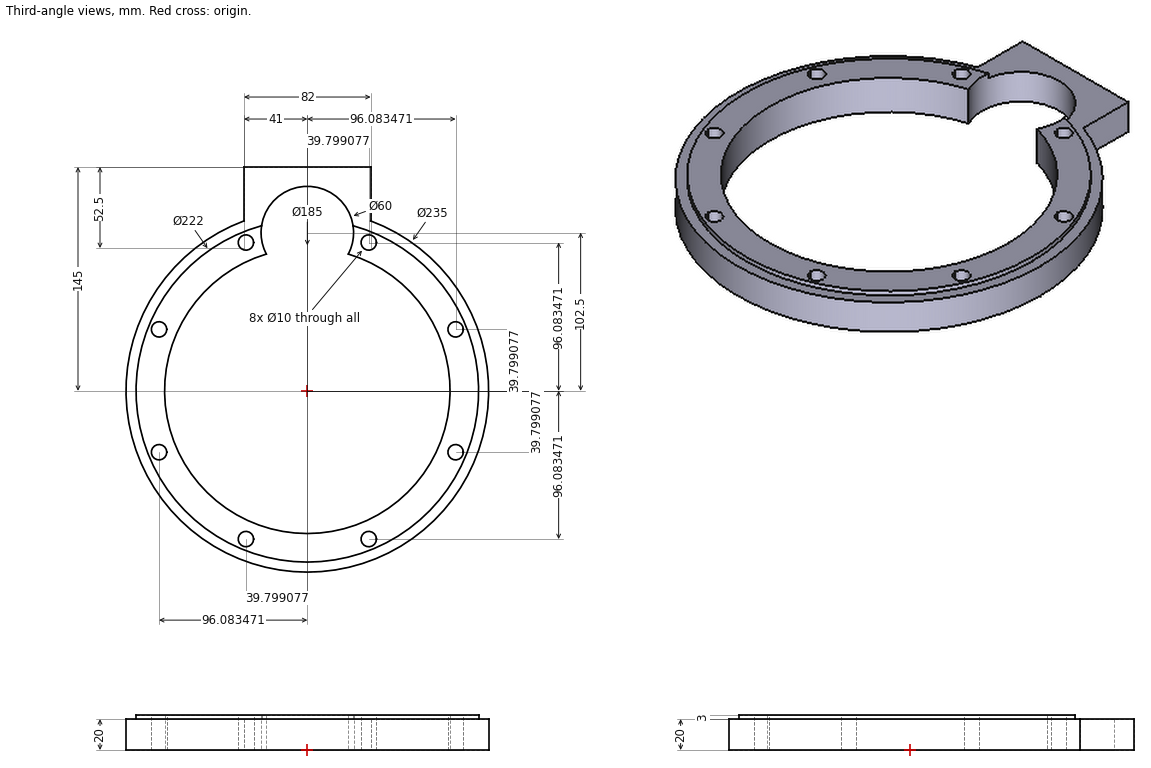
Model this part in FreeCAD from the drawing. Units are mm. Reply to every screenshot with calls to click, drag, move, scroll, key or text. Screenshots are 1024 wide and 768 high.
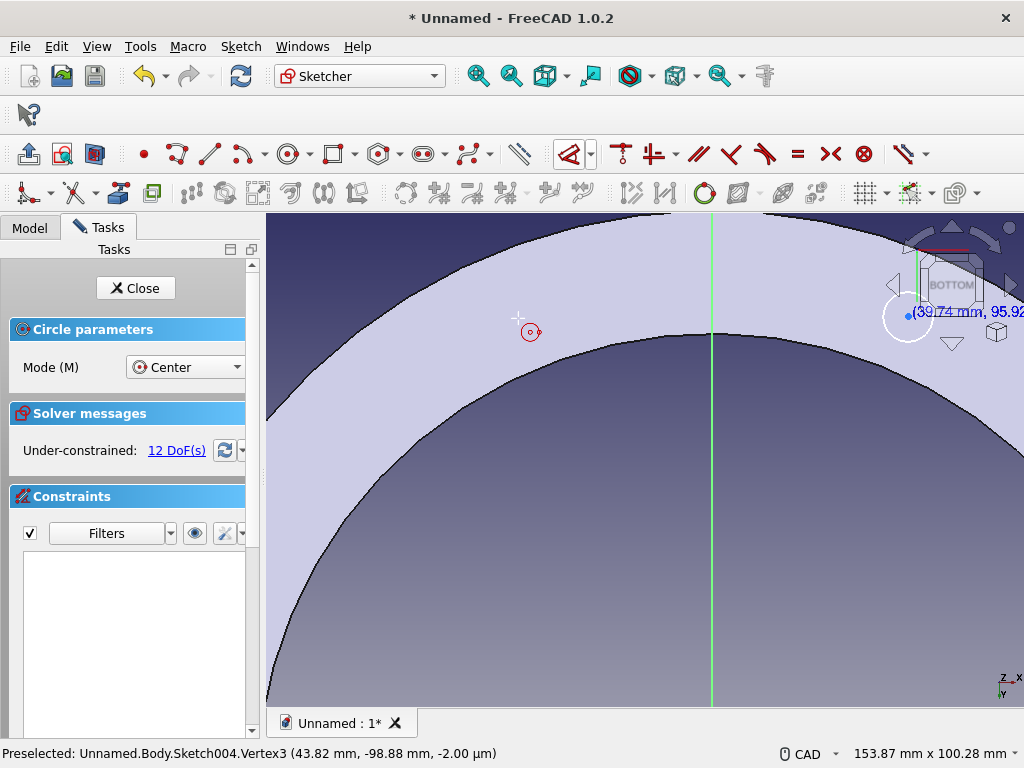
click(516, 316)
click(534, 299)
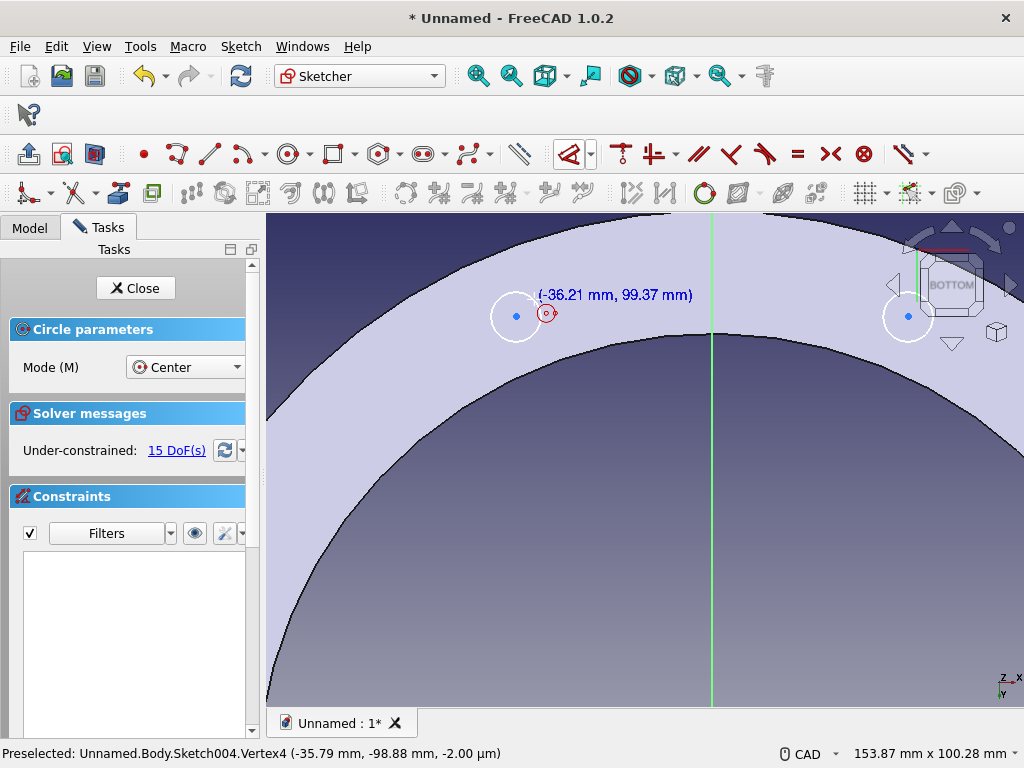
scroll(518, 318, down, 6)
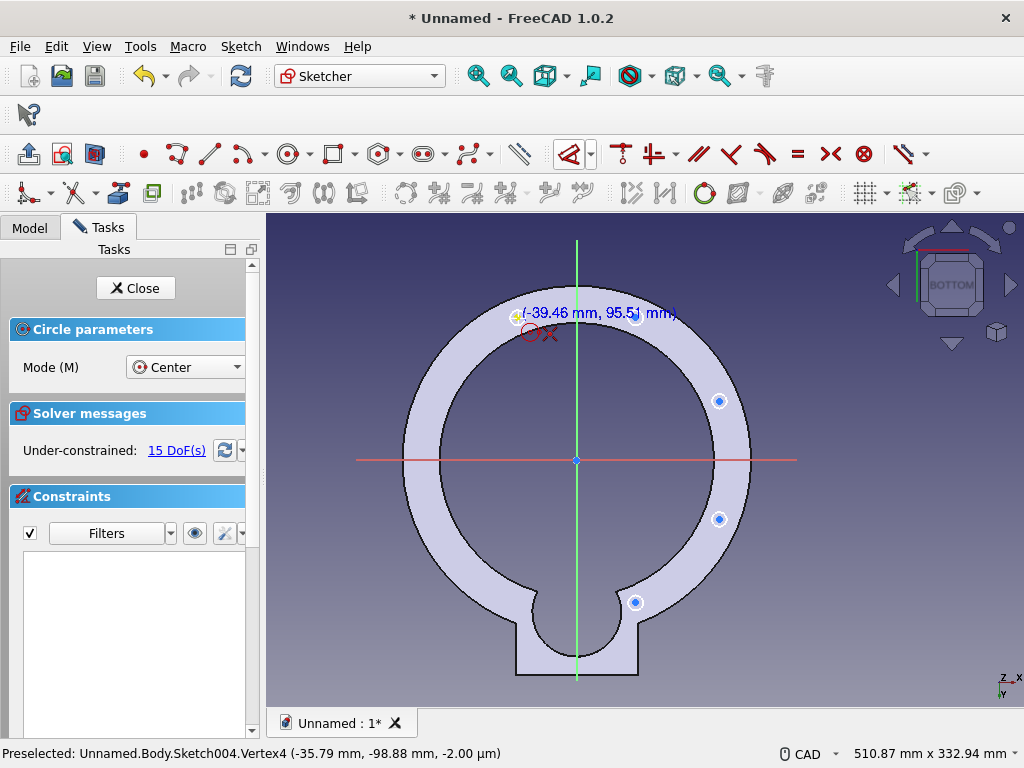
scroll(434, 401, up, 6)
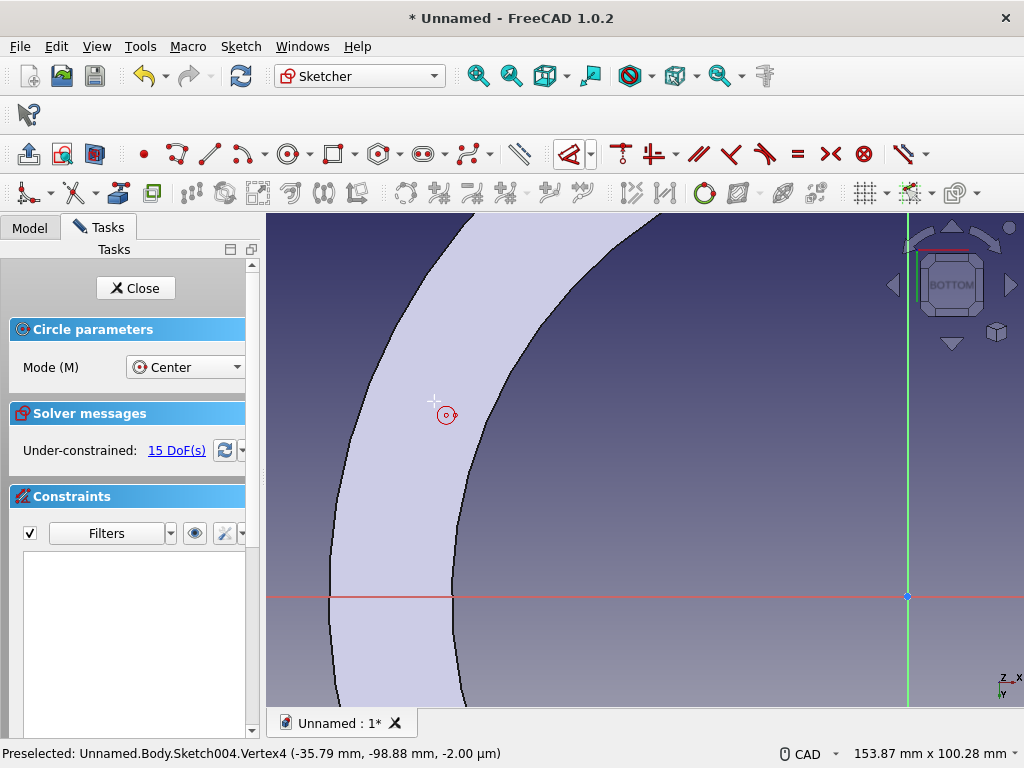
click(434, 400)
click(452, 383)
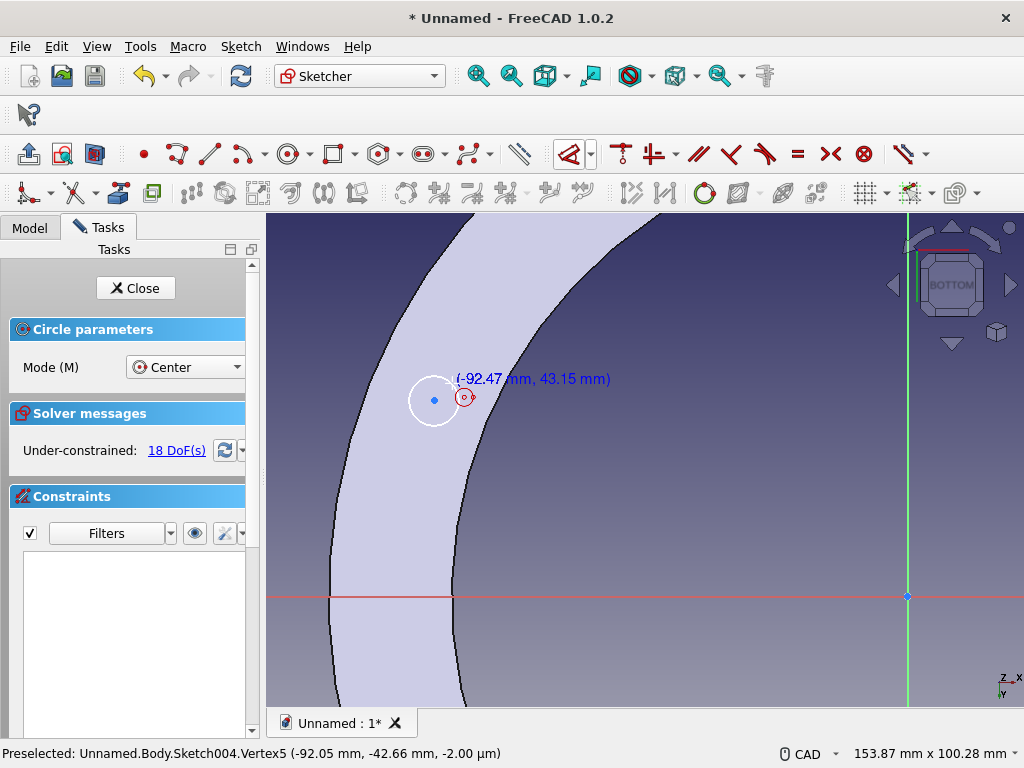
scroll(434, 401, down, 6)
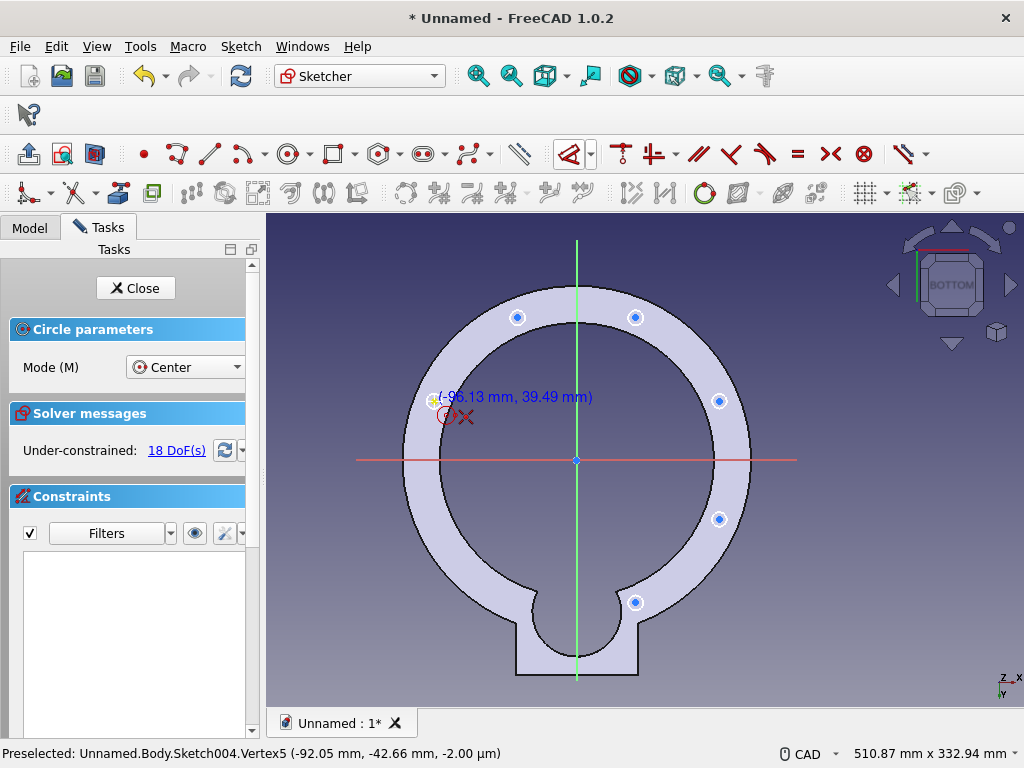
scroll(434, 519, up, 6)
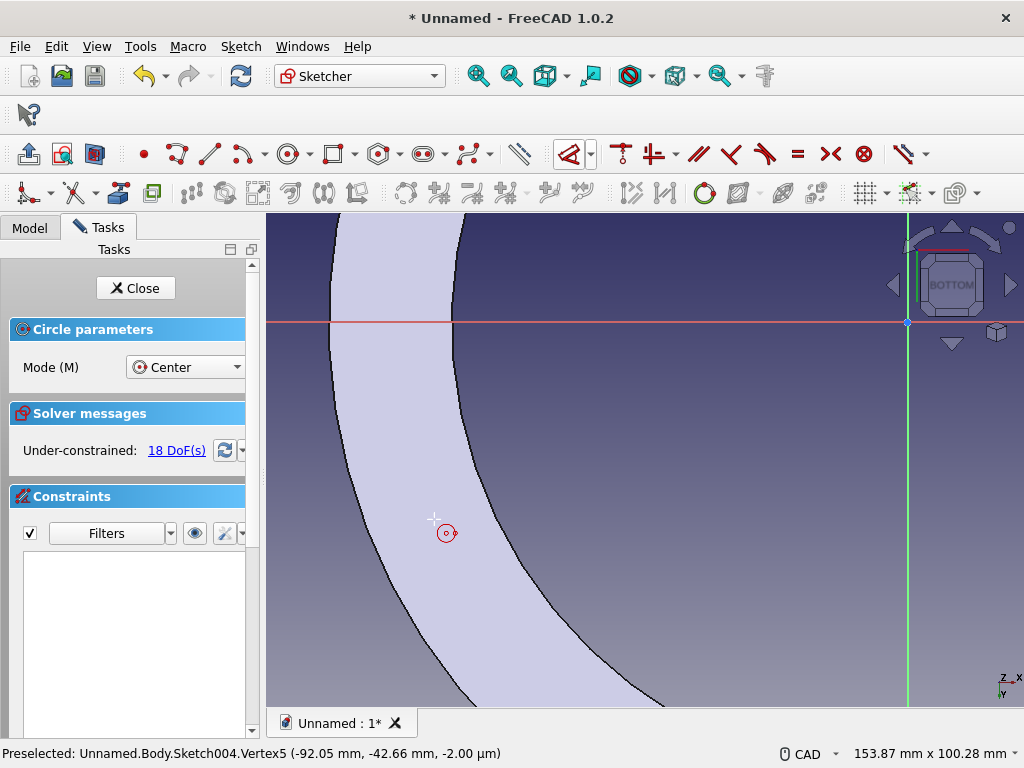
click(434, 518)
click(452, 501)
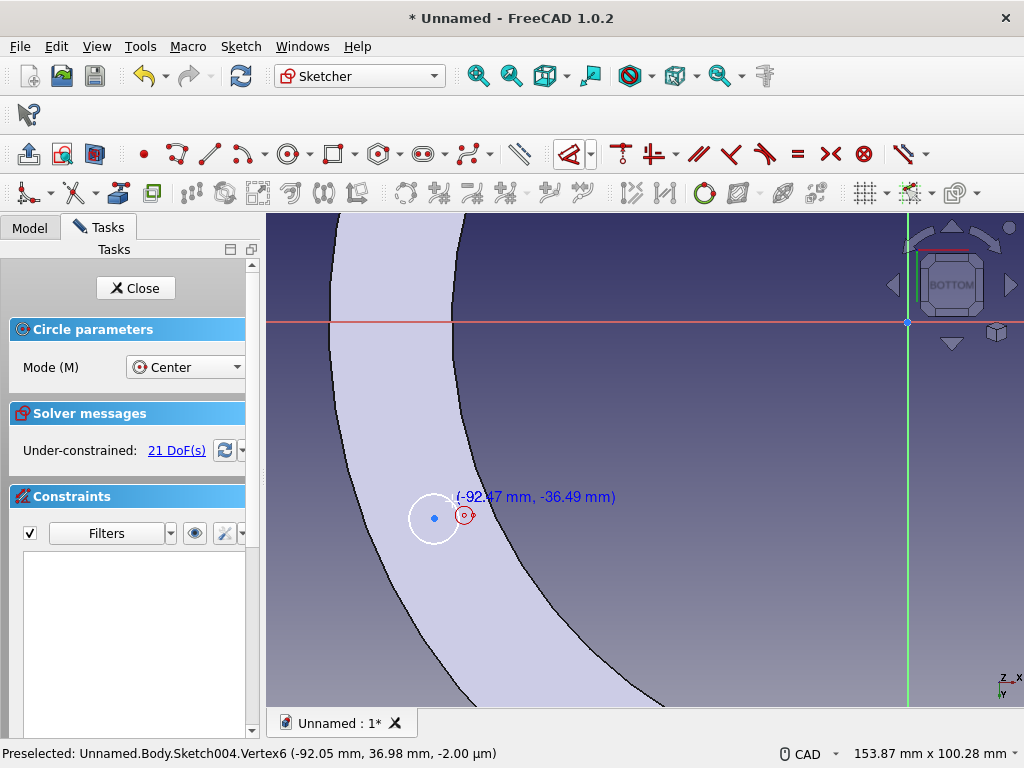
scroll(434, 519, down, 6)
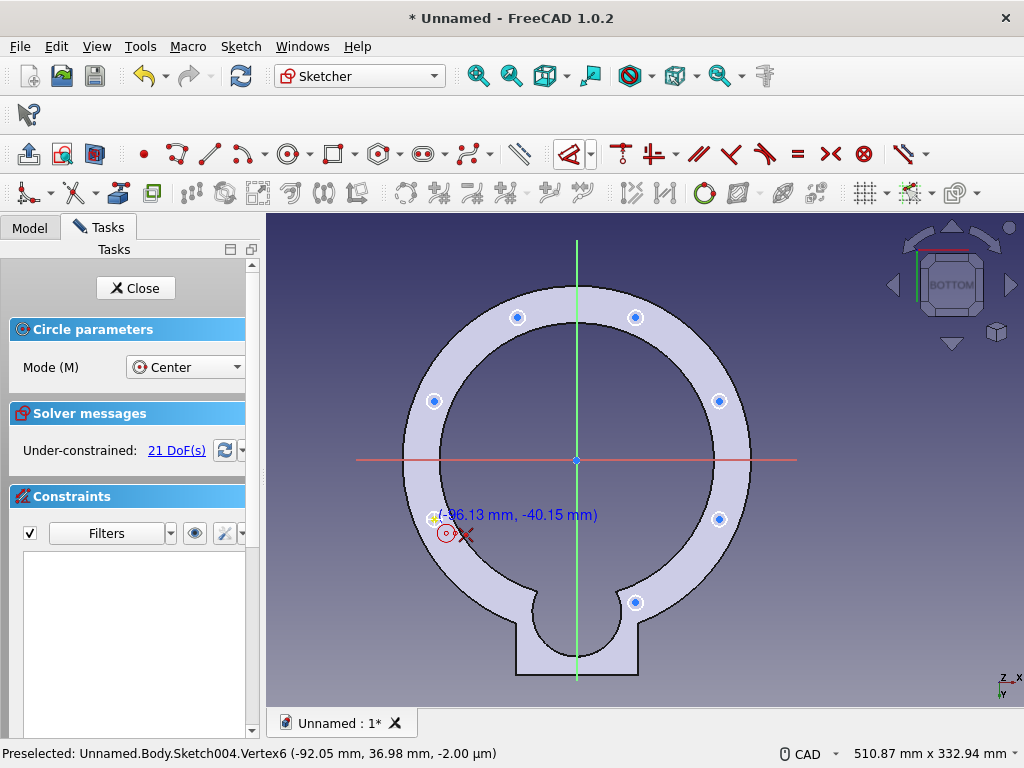
scroll(518, 603, up, 6)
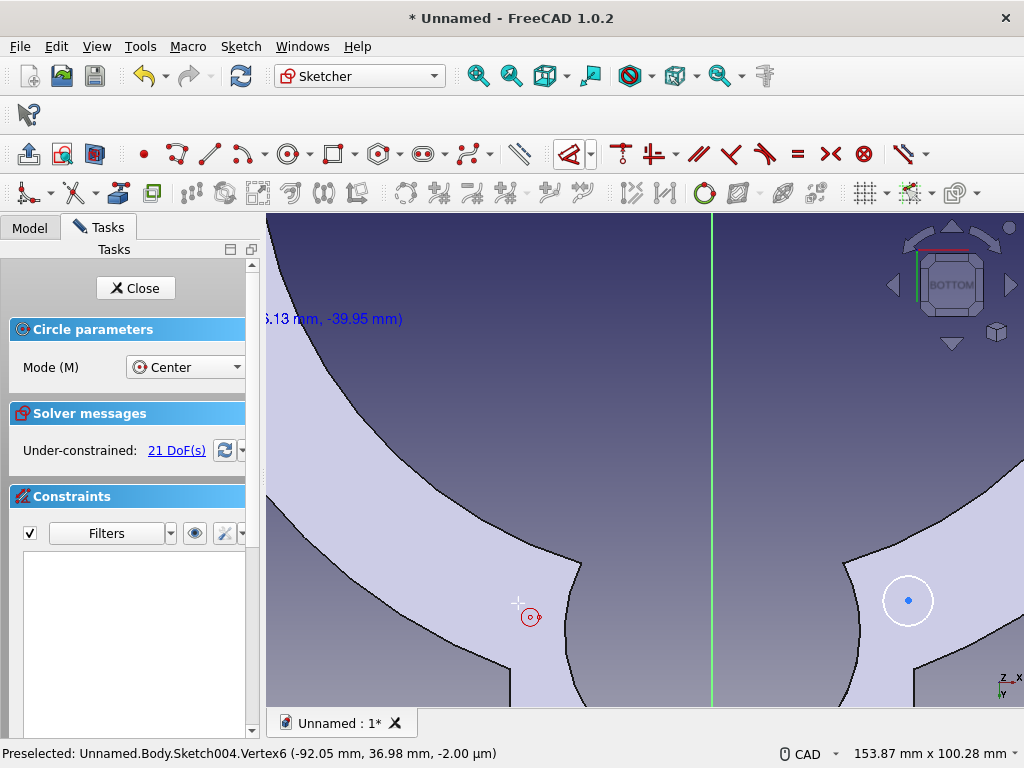
click(516, 600)
click(534, 583)
key(Escape)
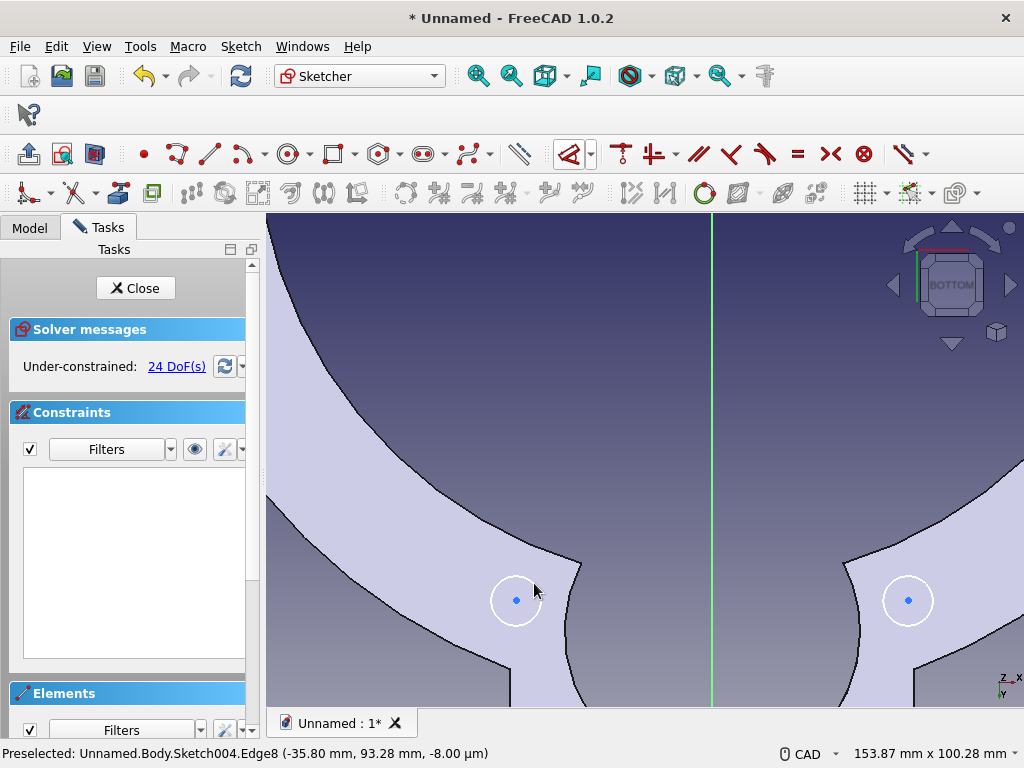
scroll(518, 604, down, 6)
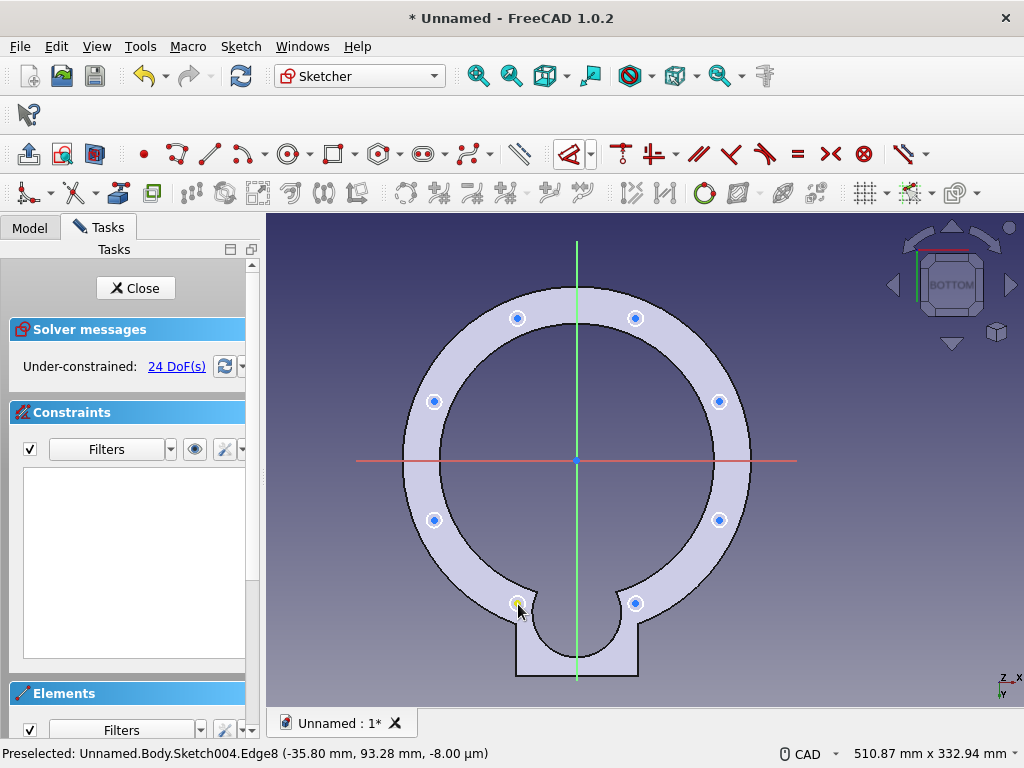
scroll(641, 598, up, 4)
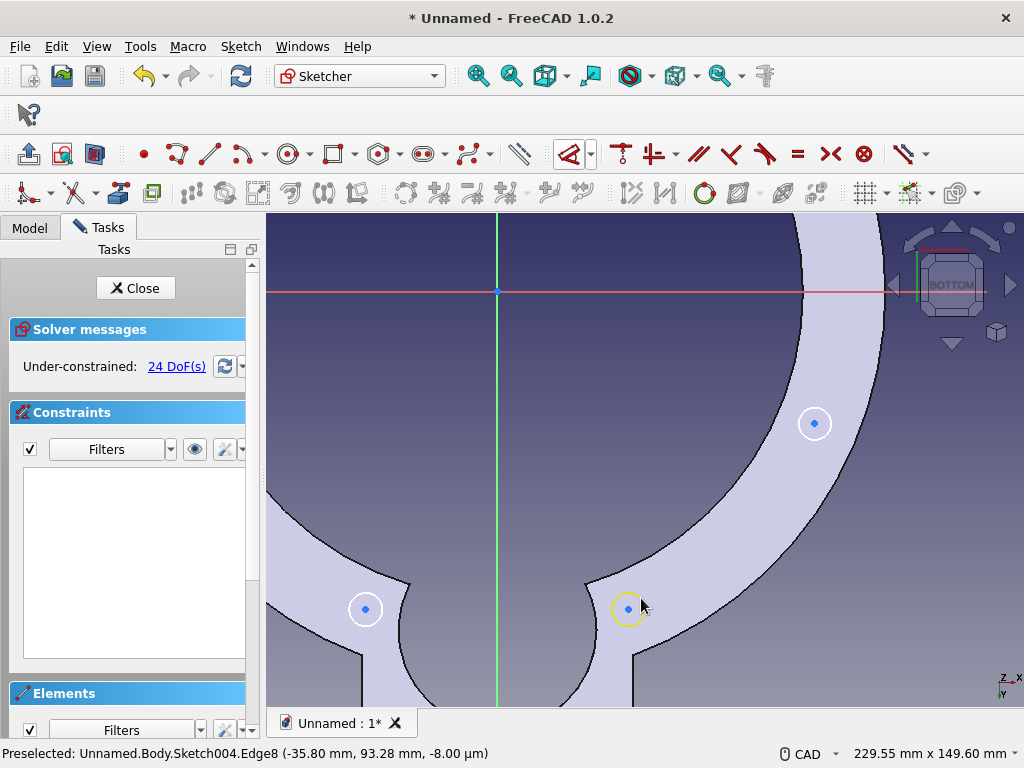
click(640, 598)